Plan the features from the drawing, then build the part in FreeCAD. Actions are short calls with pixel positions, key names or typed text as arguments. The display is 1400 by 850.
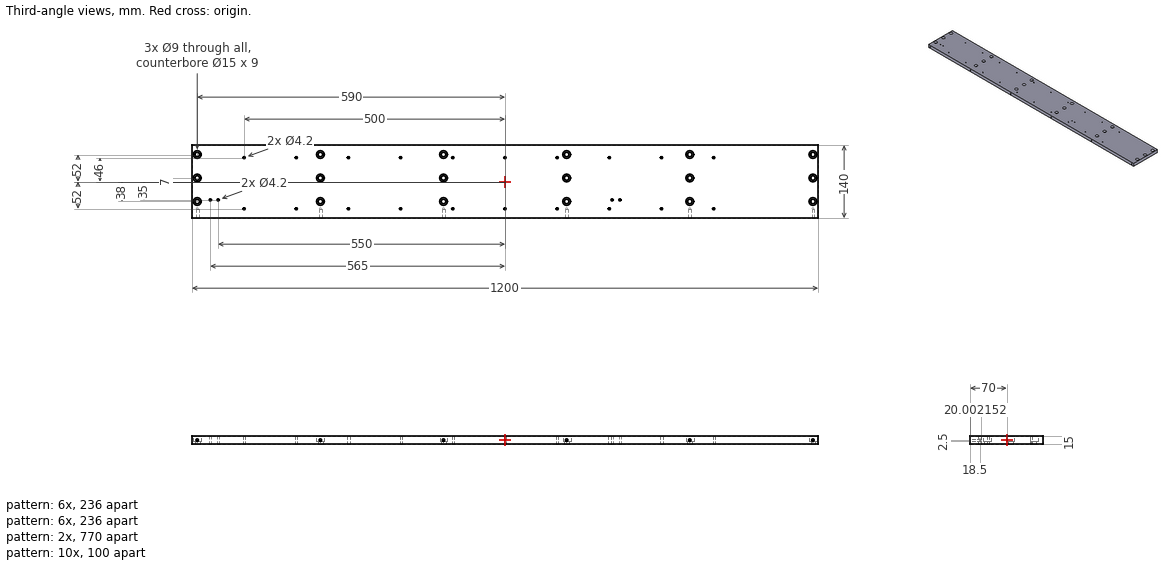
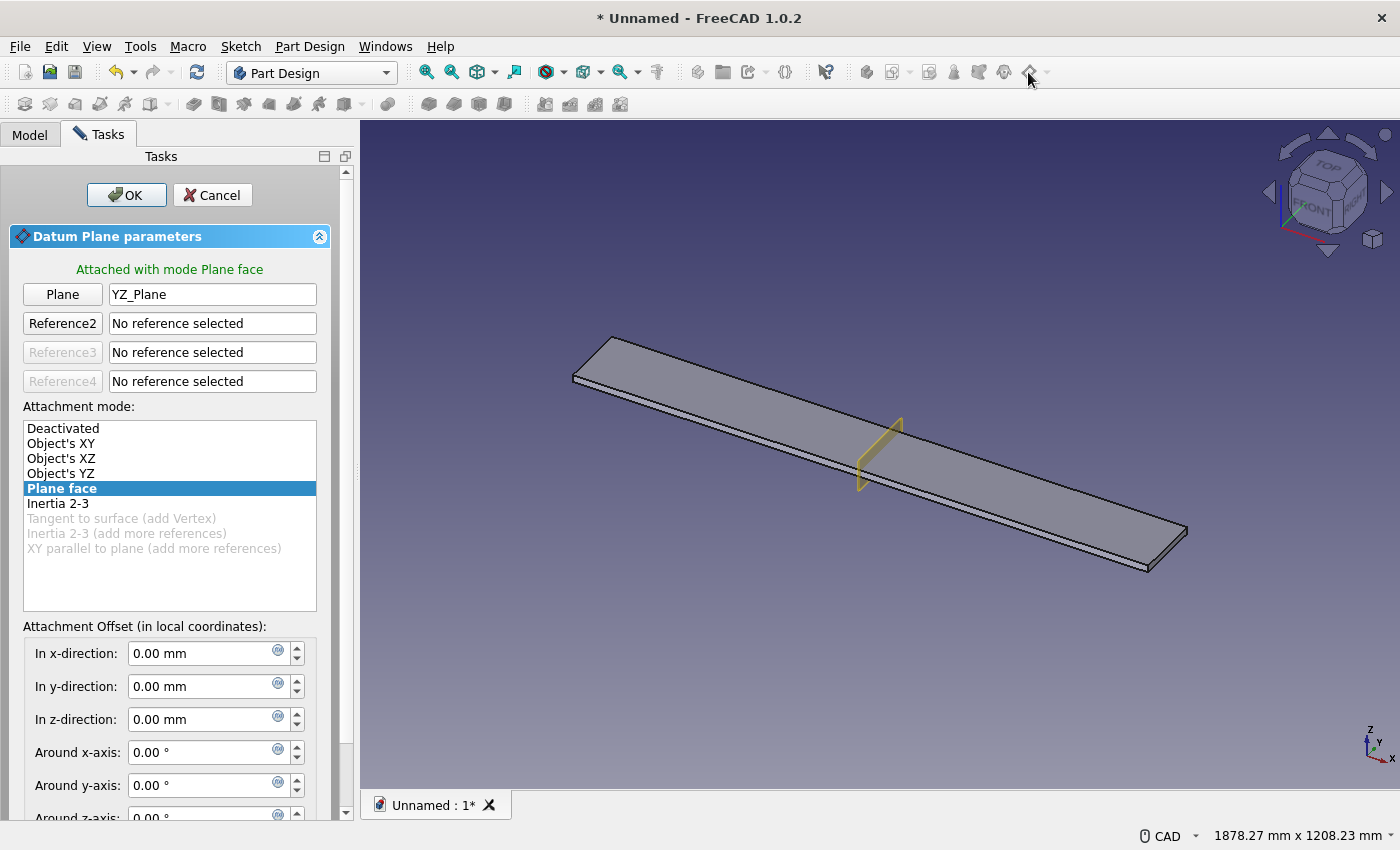
triple_click(210, 720)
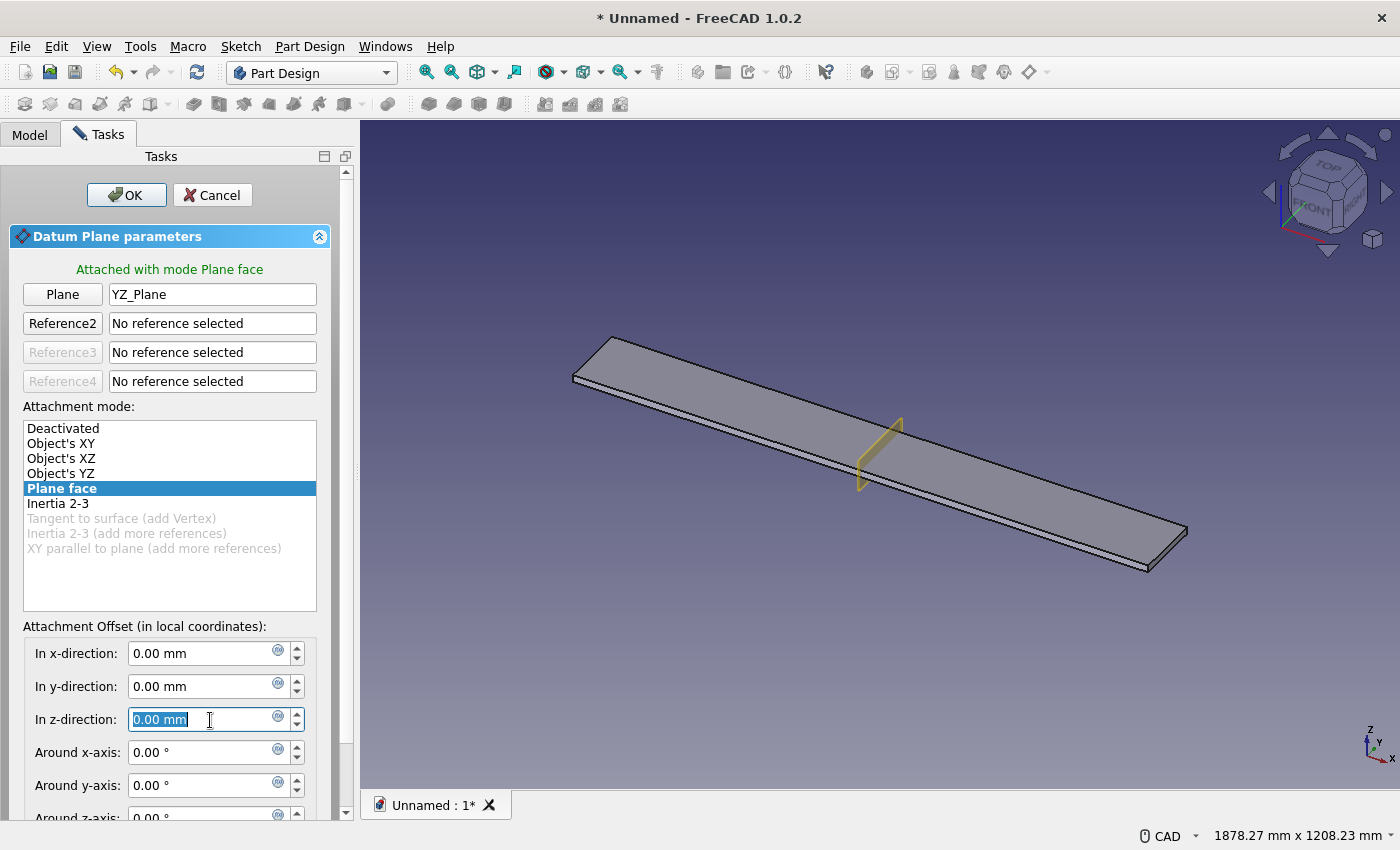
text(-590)
key(Tab)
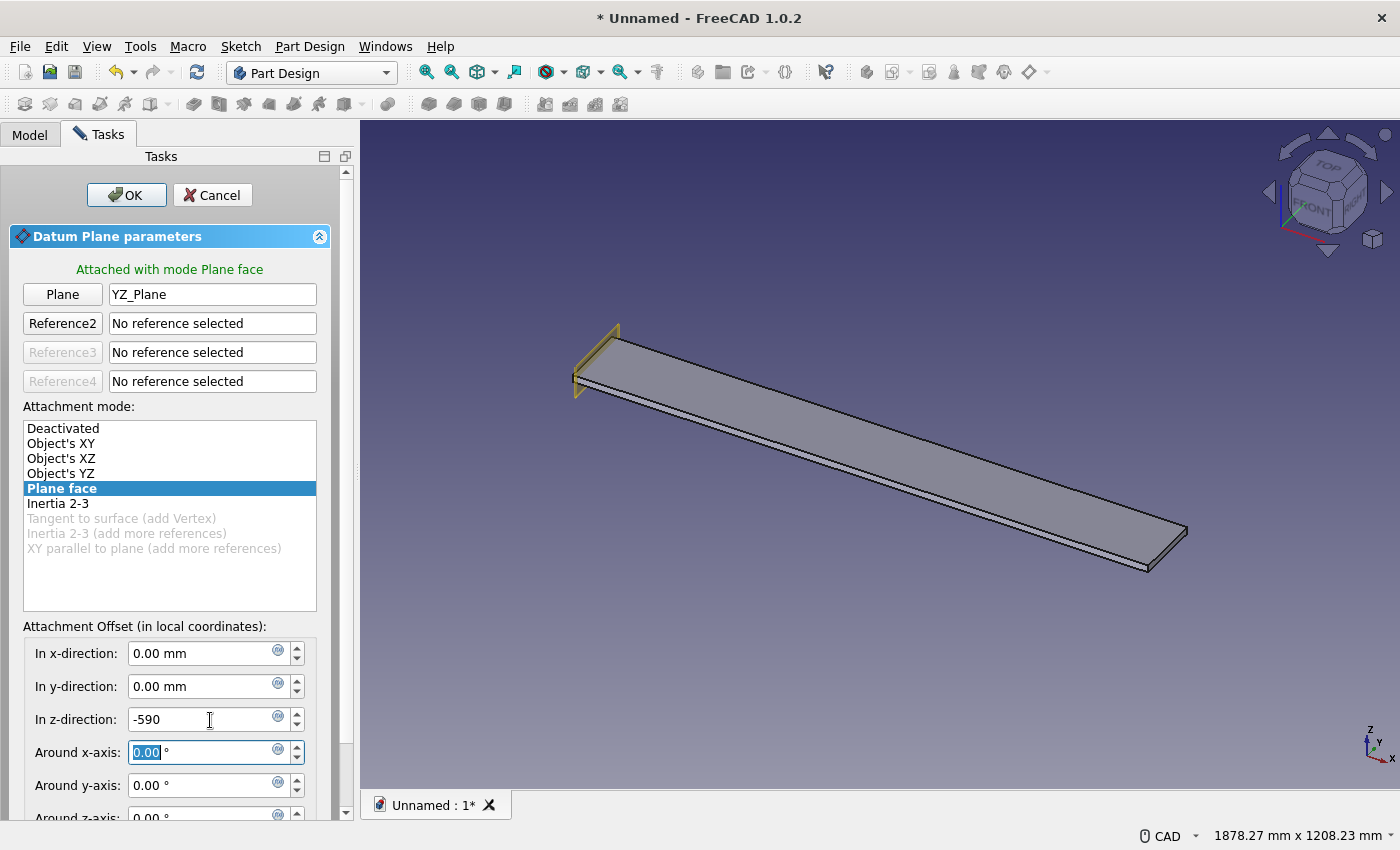
click(127, 195)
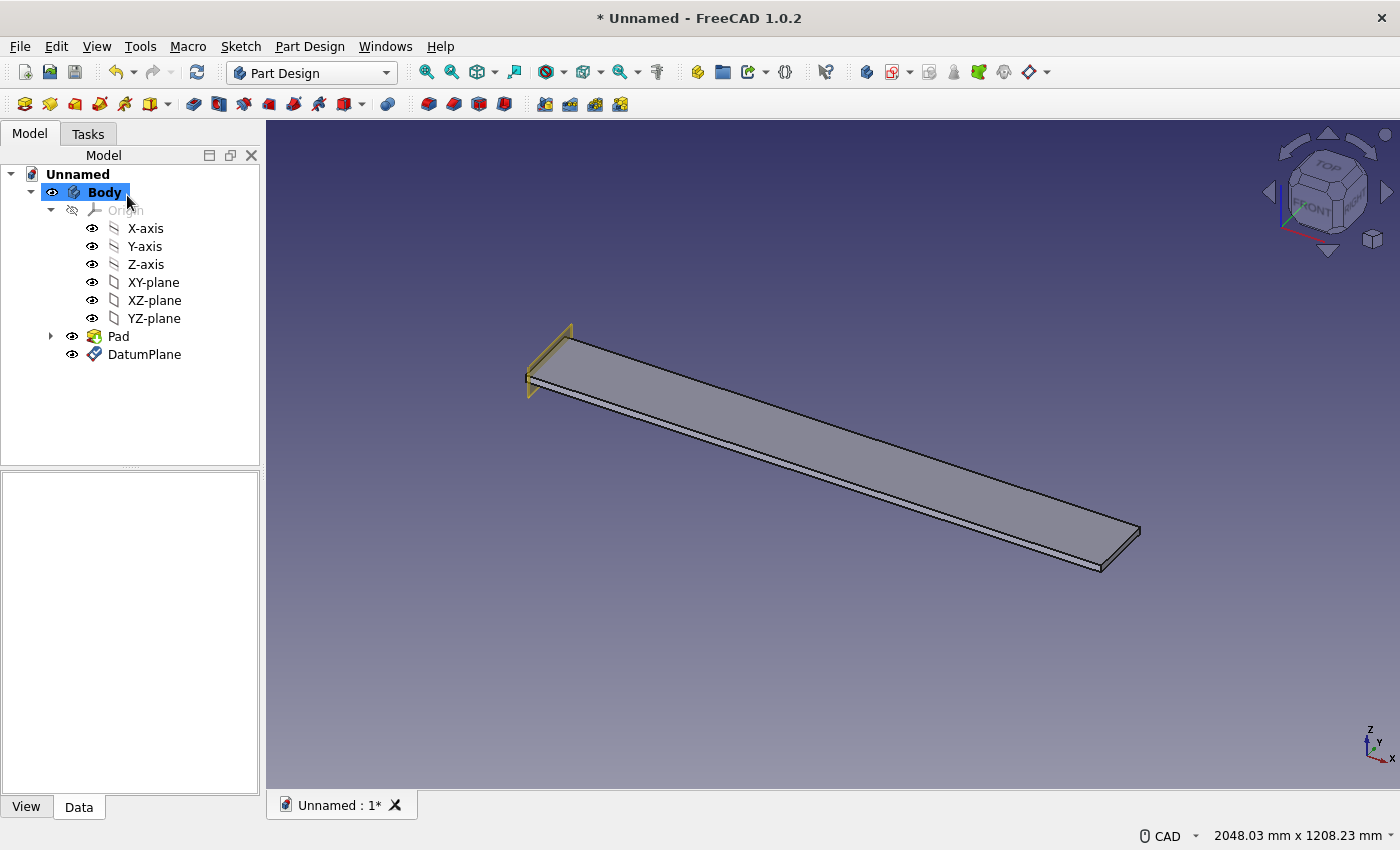
click(117, 354)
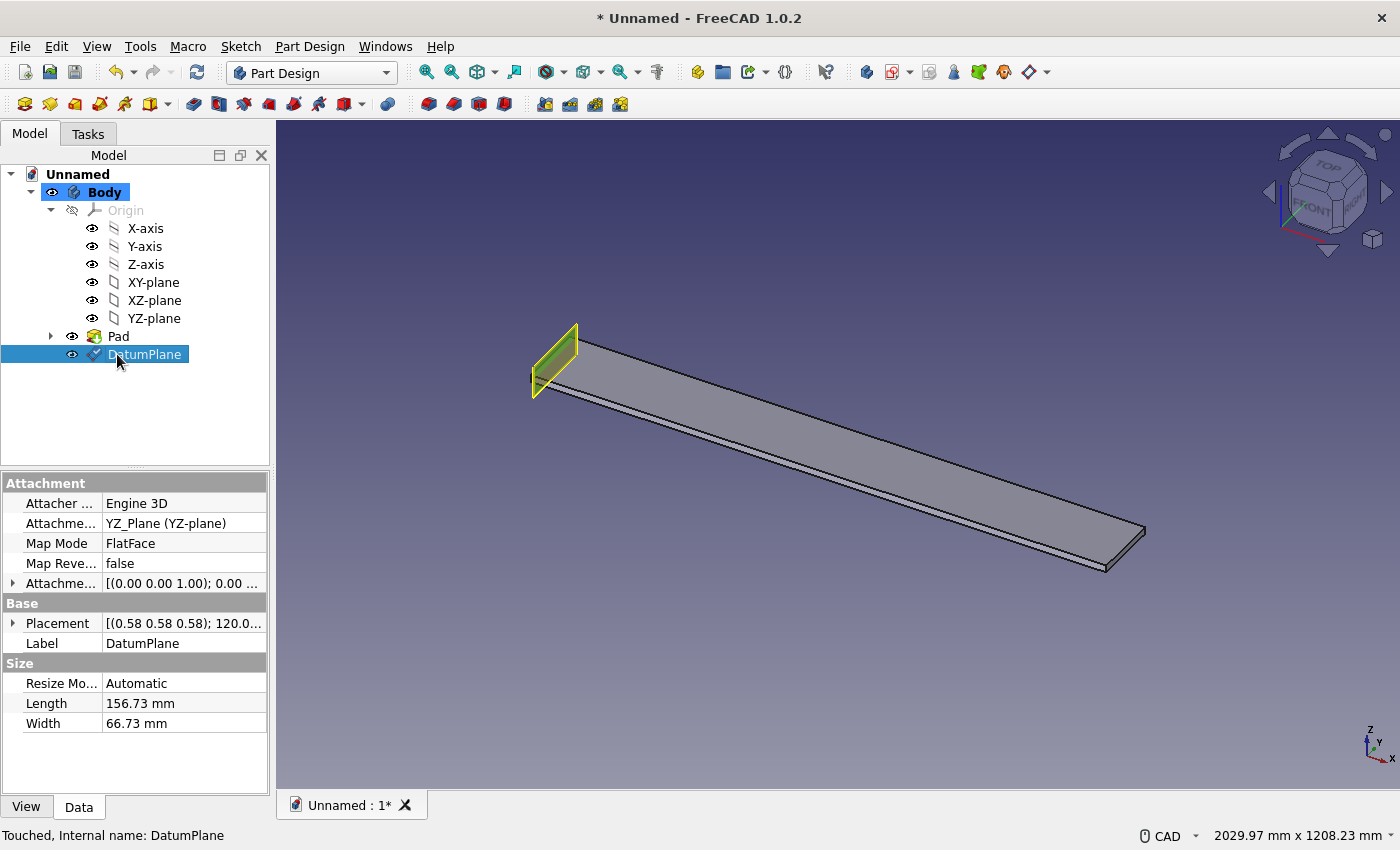
click(892, 72)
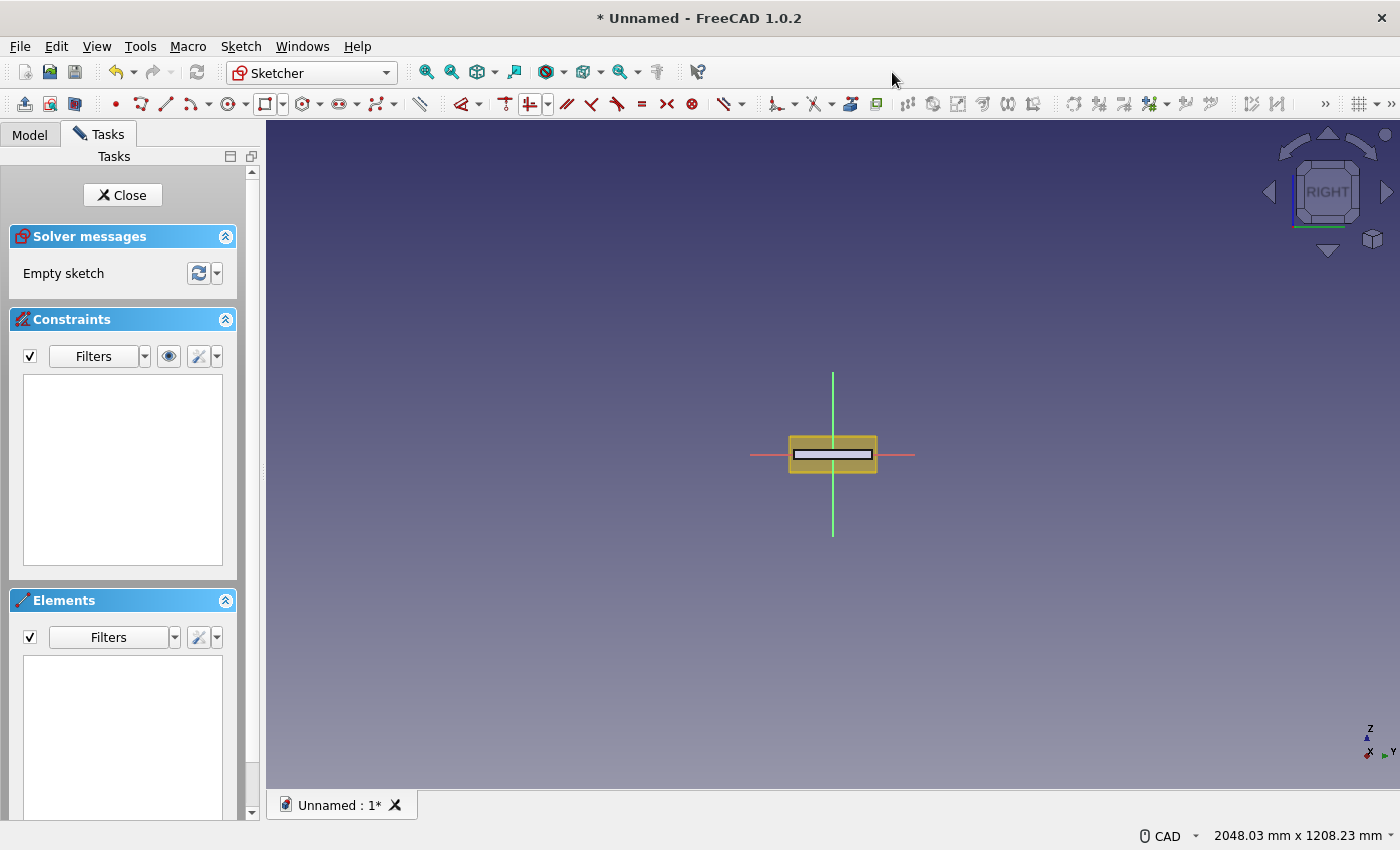
key(q)
key(s)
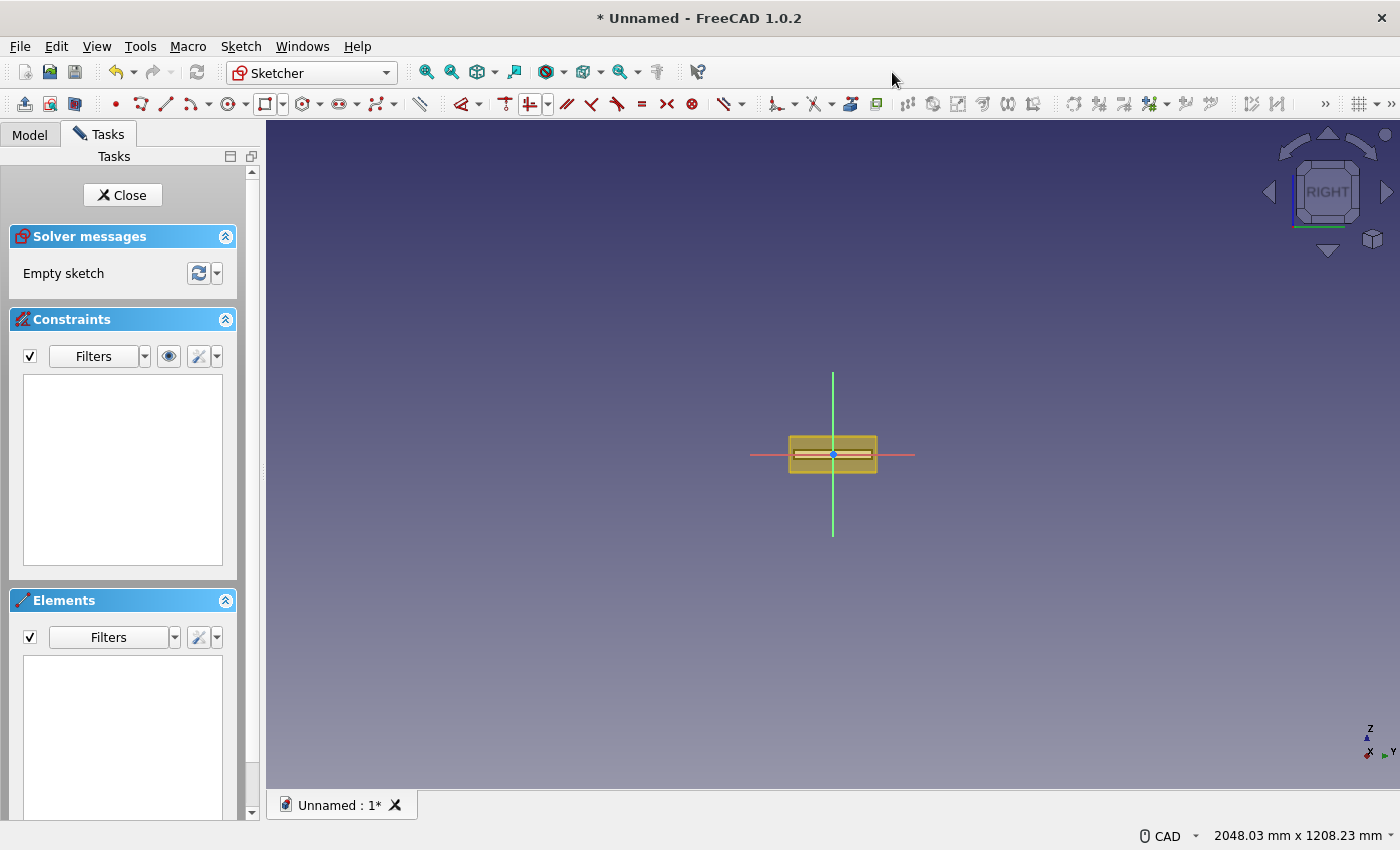
scroll(802, 455, up, 15)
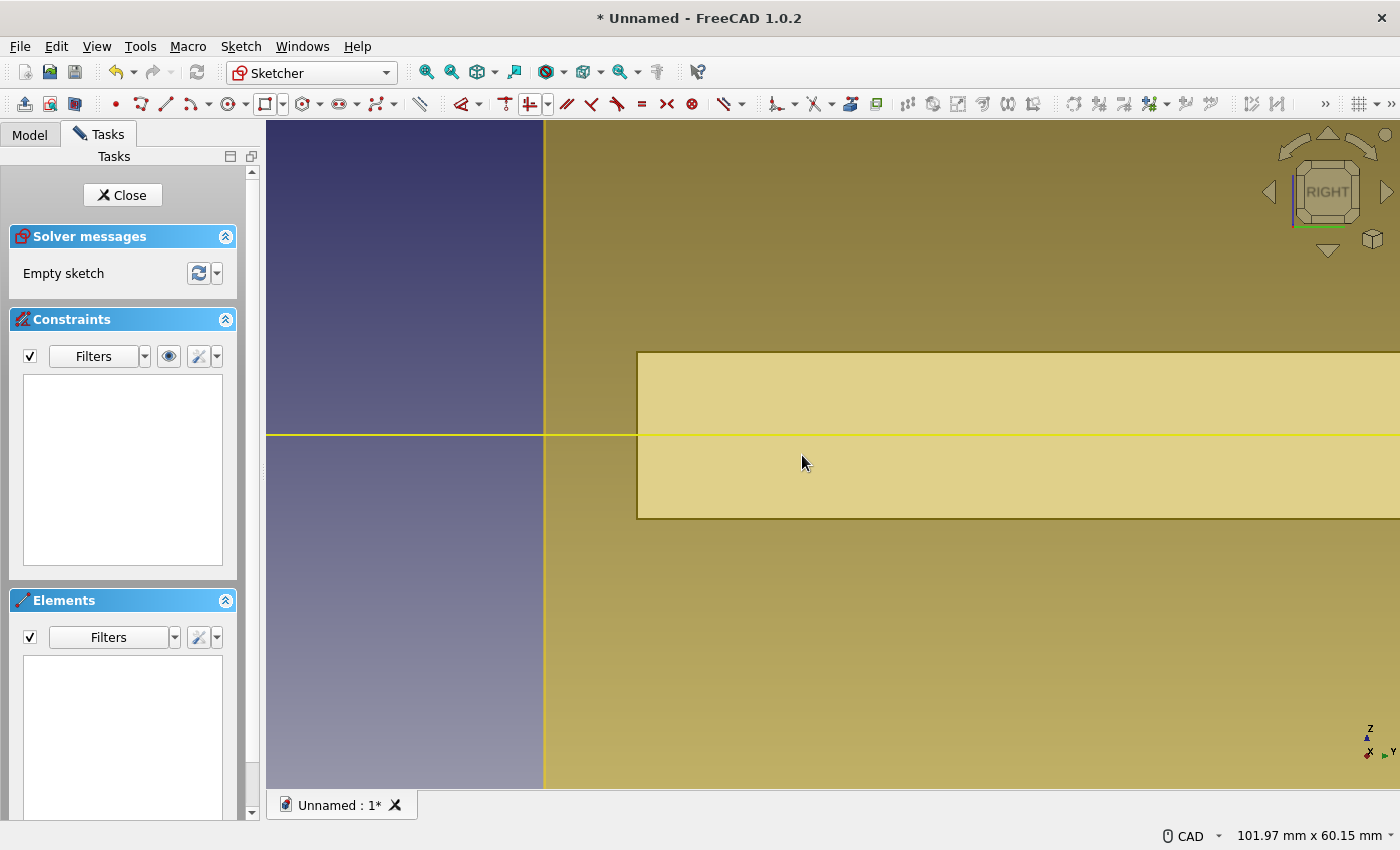
scroll(739, 446, up, 5)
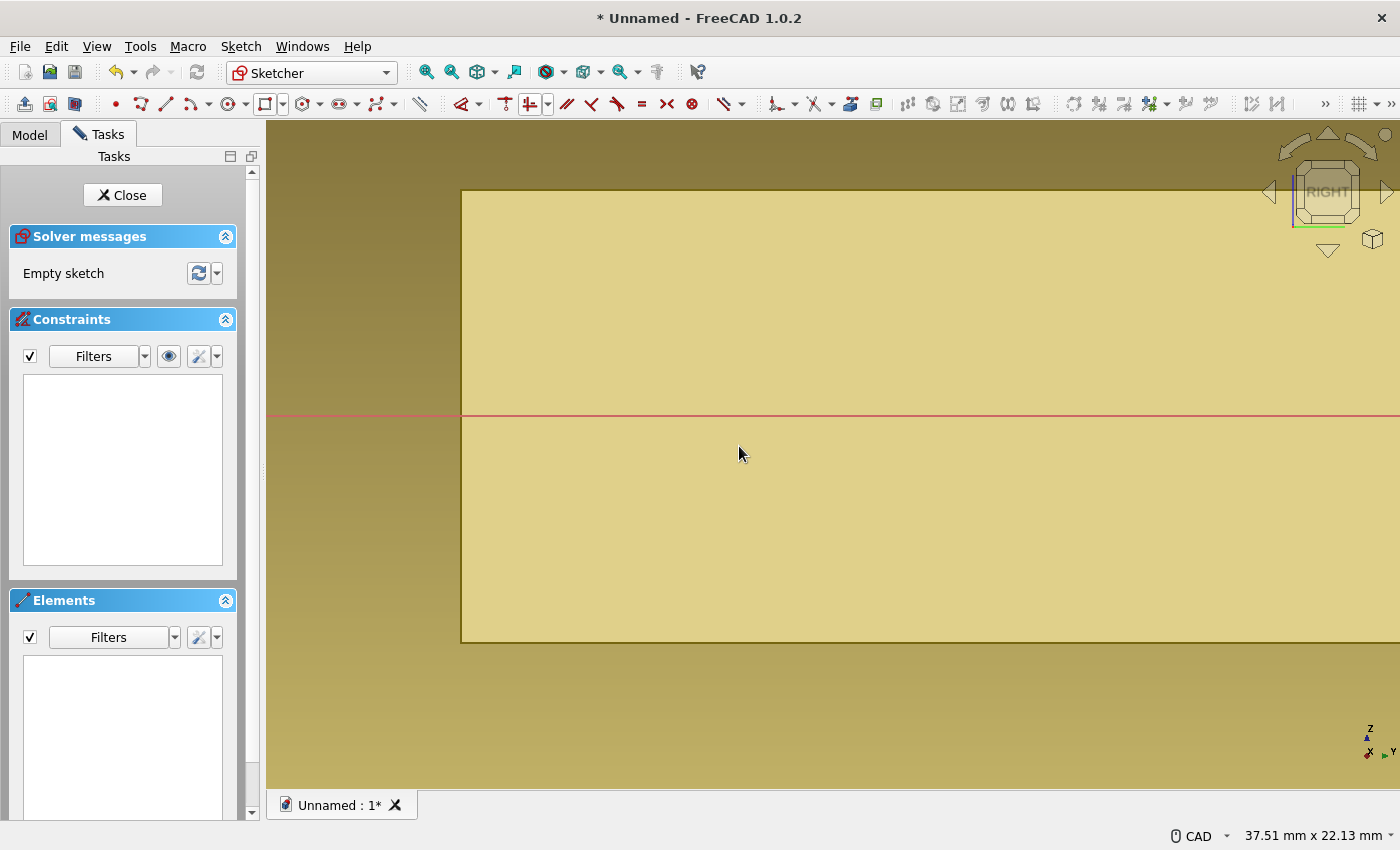
key(g)
key(m)